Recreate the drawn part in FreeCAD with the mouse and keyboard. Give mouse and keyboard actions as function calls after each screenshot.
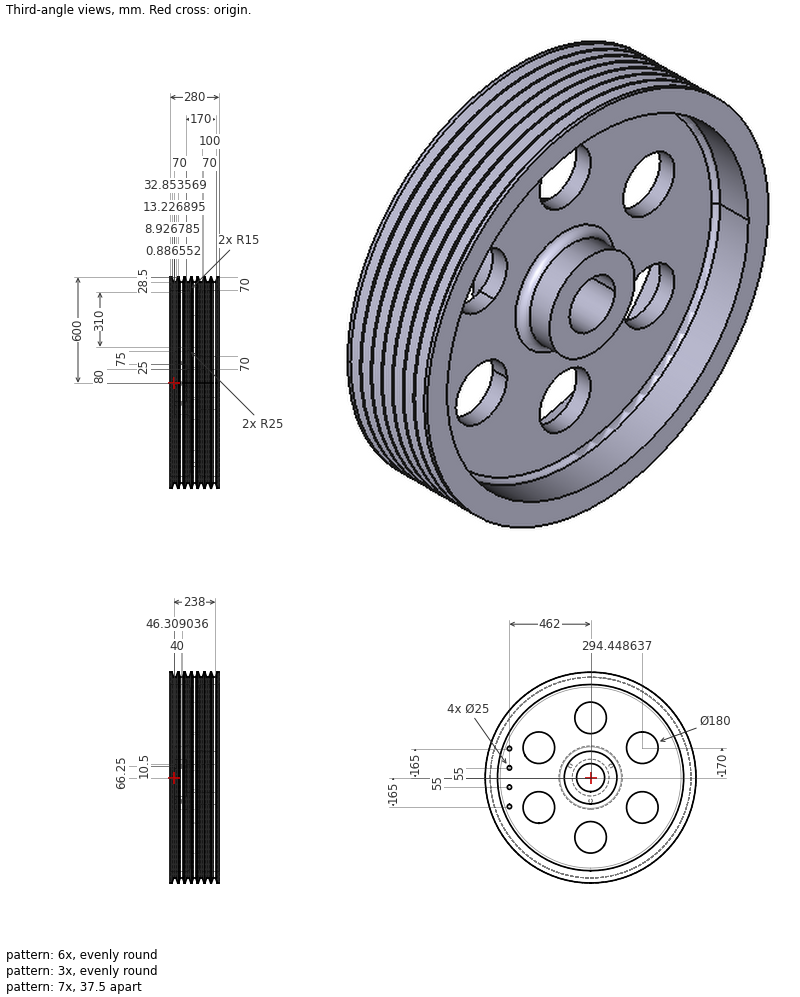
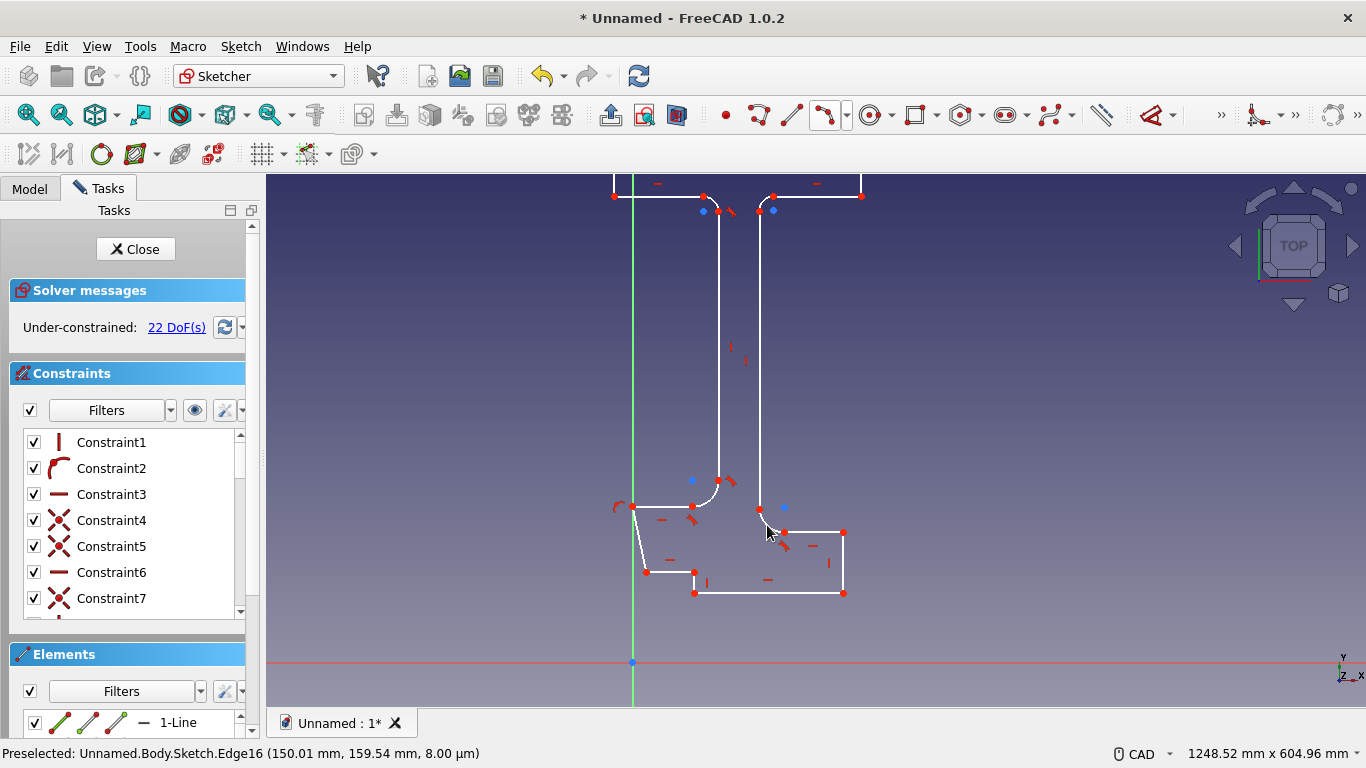
click(760, 420)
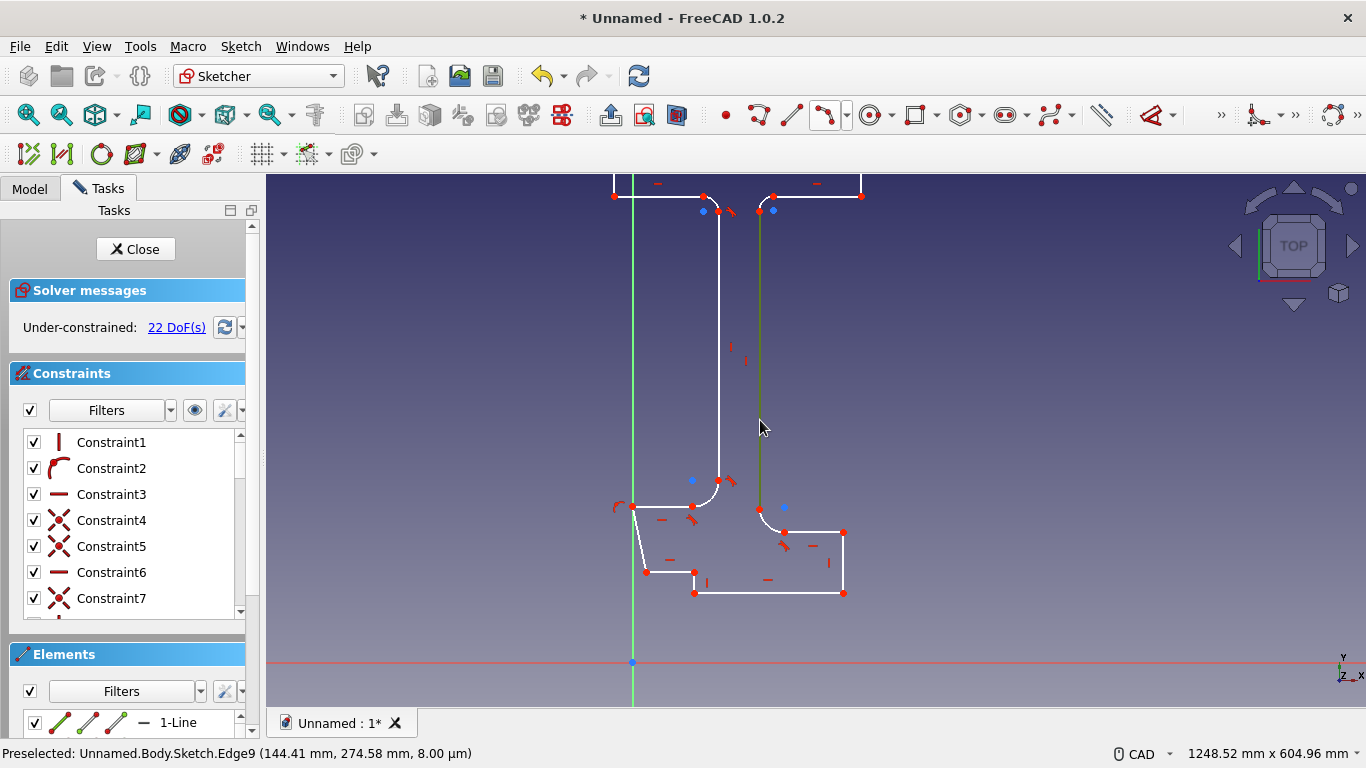
scroll(763, 520, up, 2)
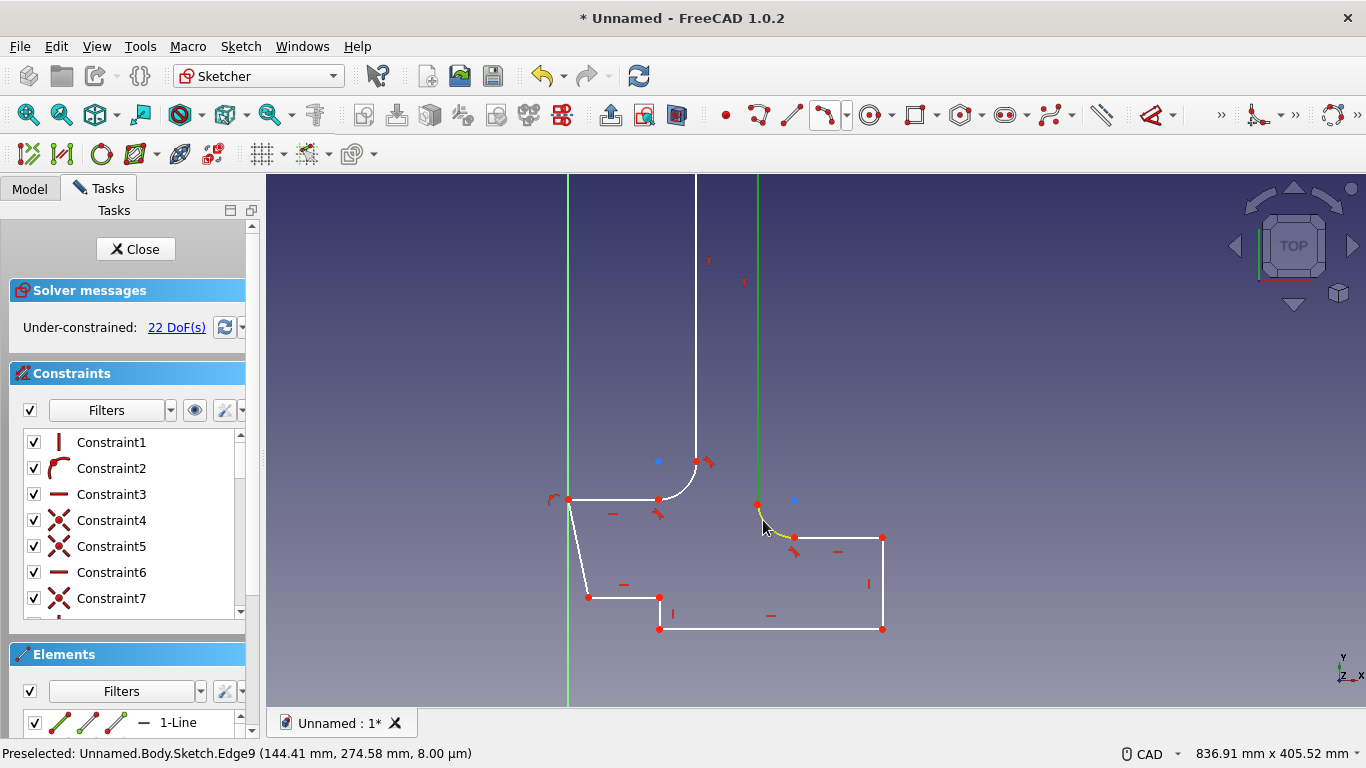
click(763, 520)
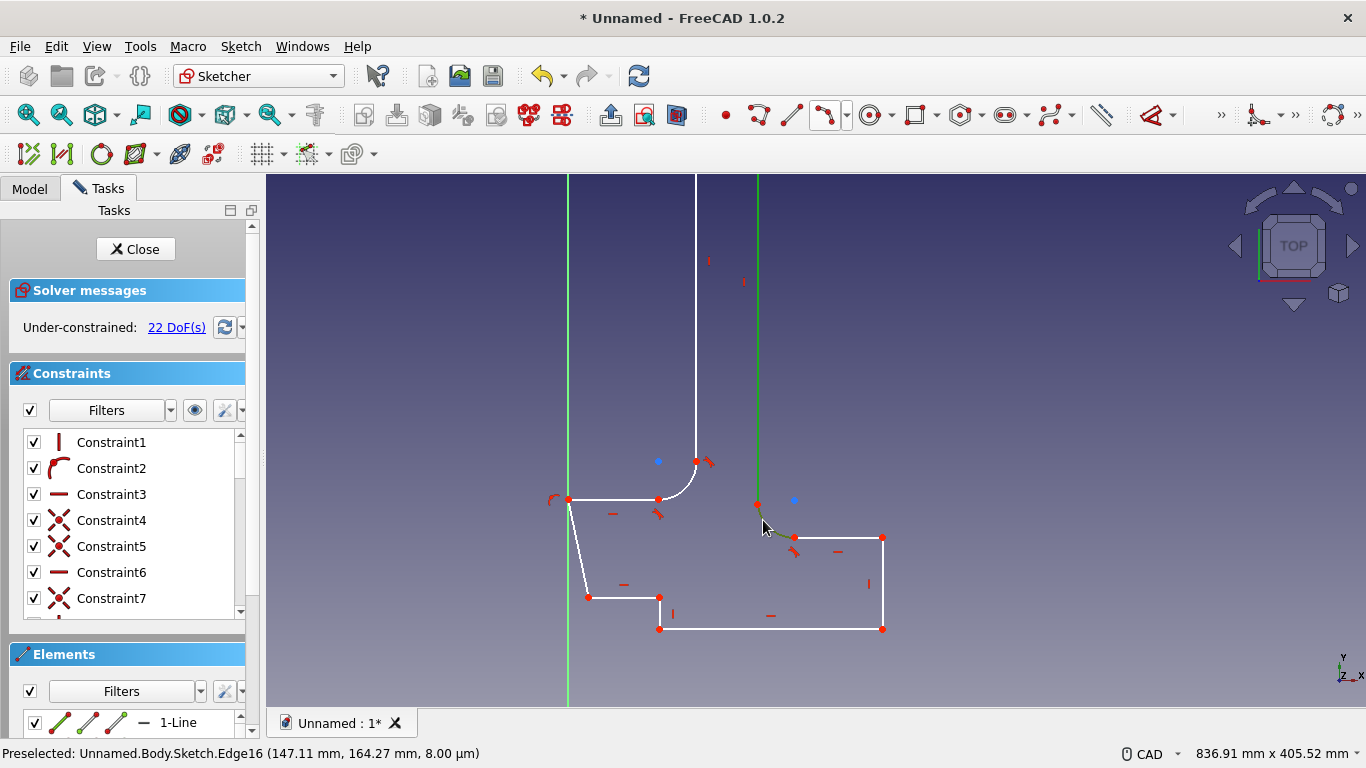
key(t)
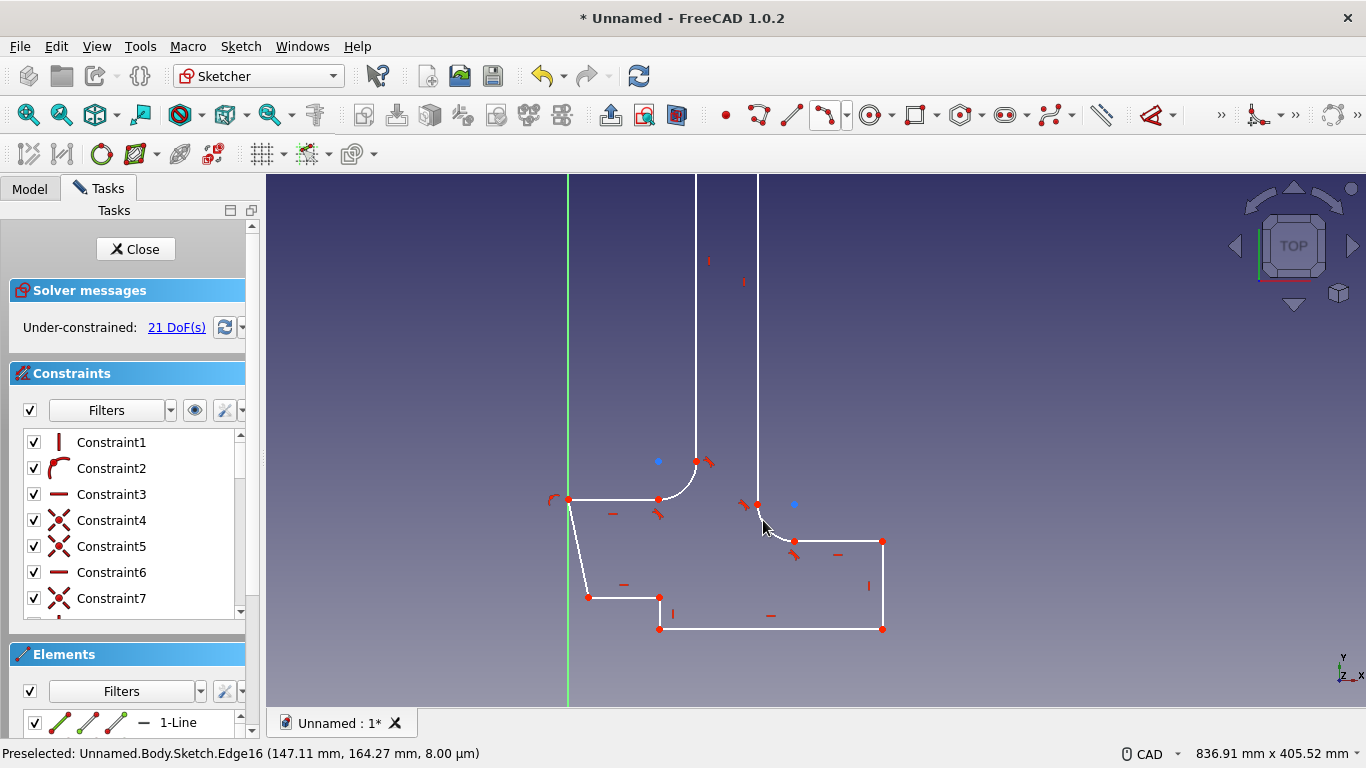
click(758, 371)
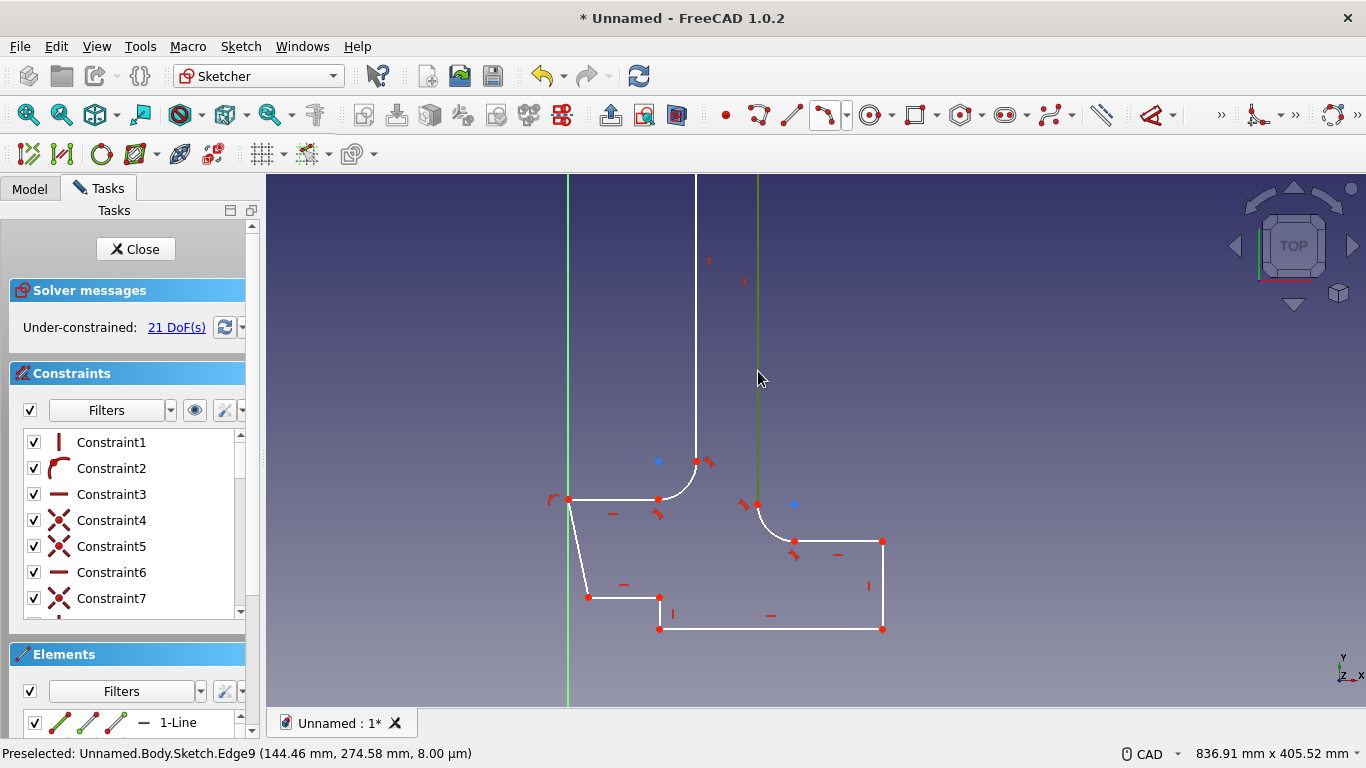
scroll(765, 524, down, 4)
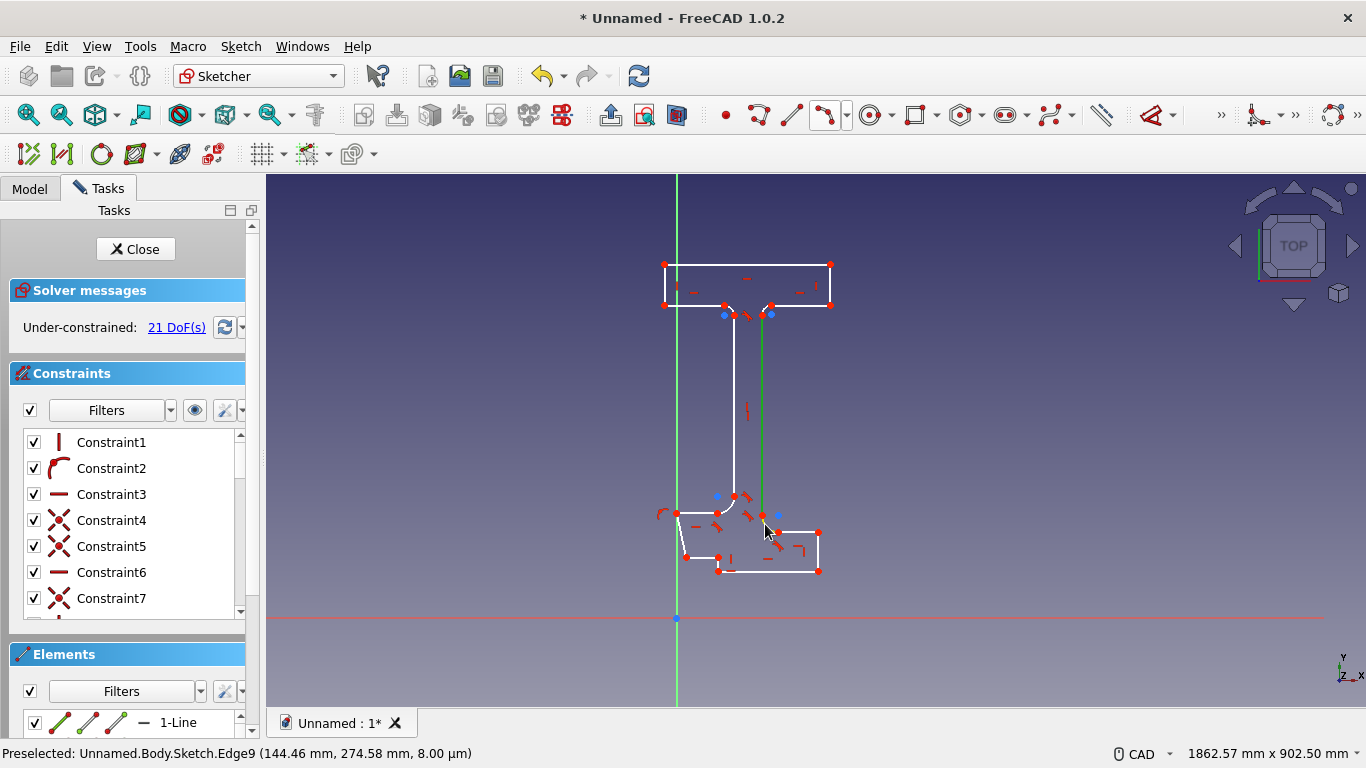
scroll(767, 307, up, 6)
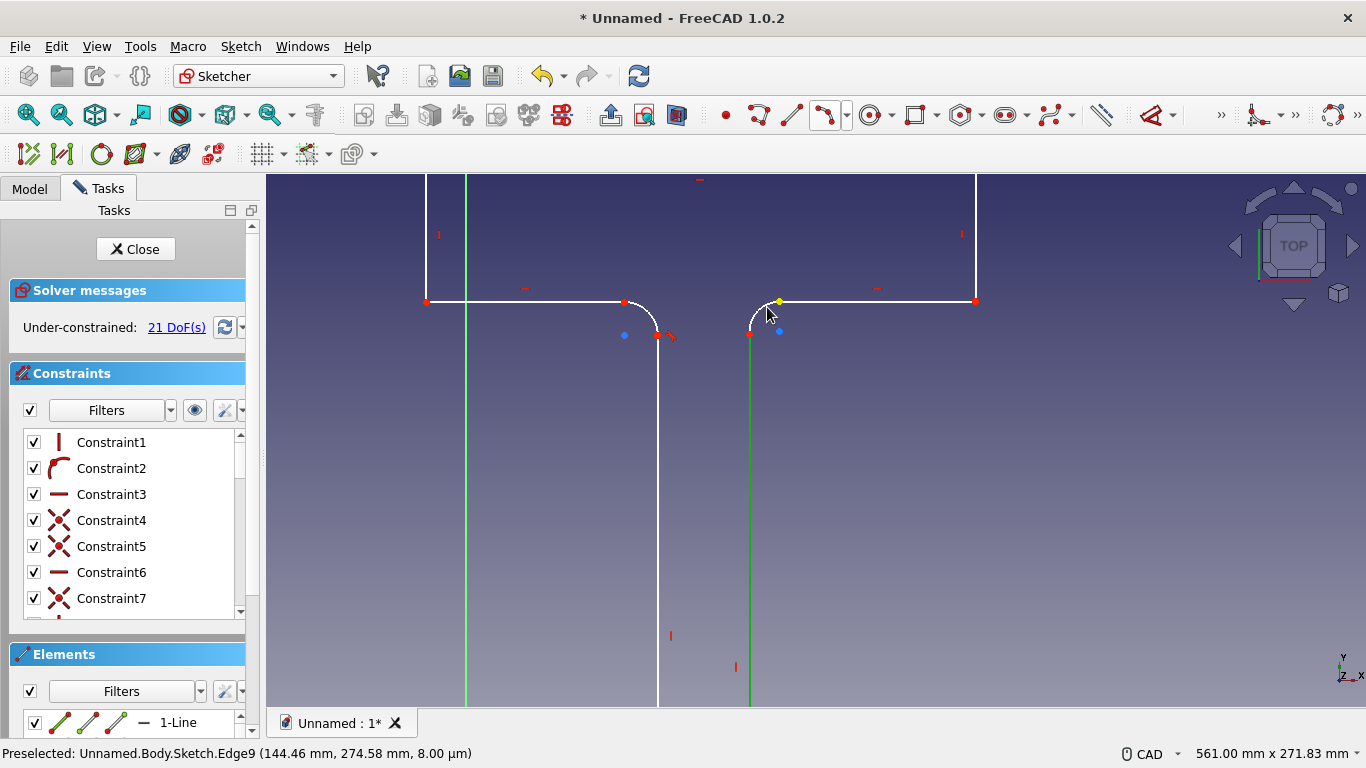
click(765, 305)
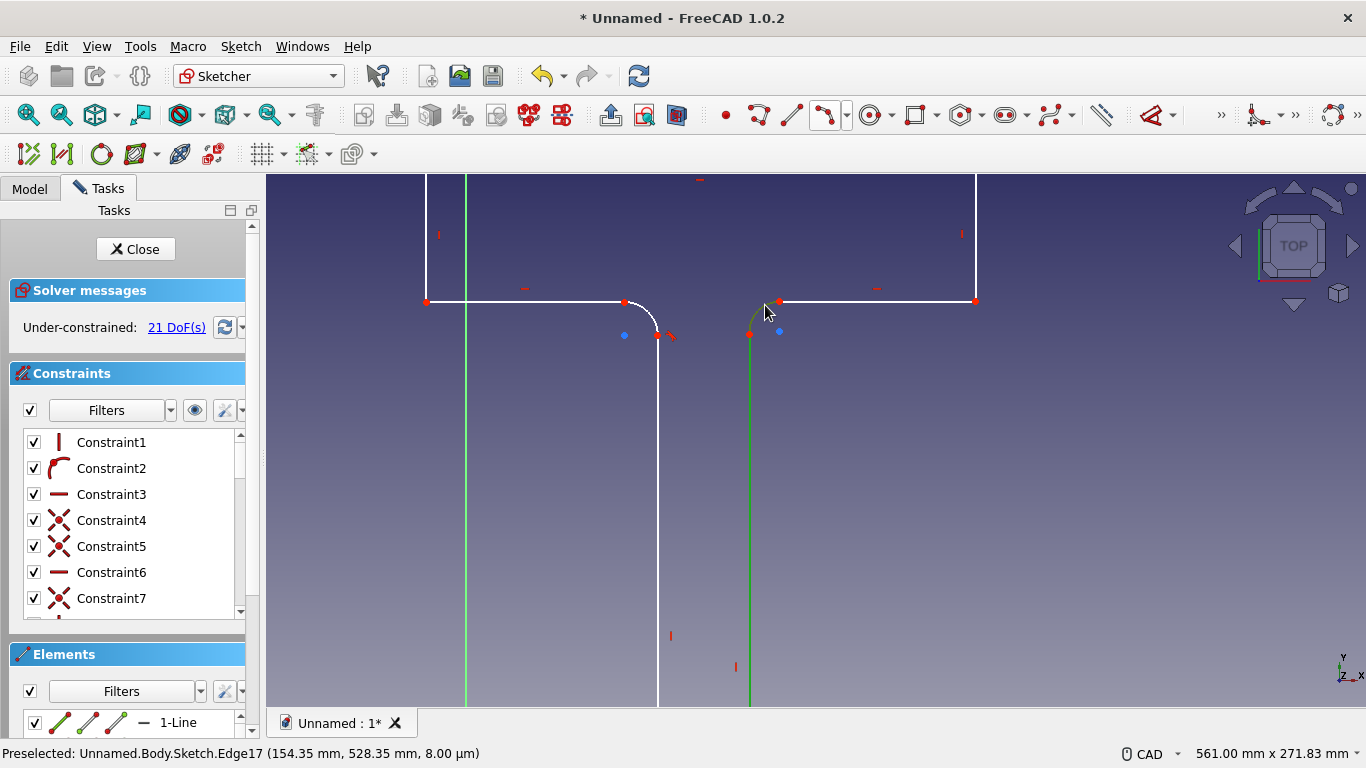
key(t)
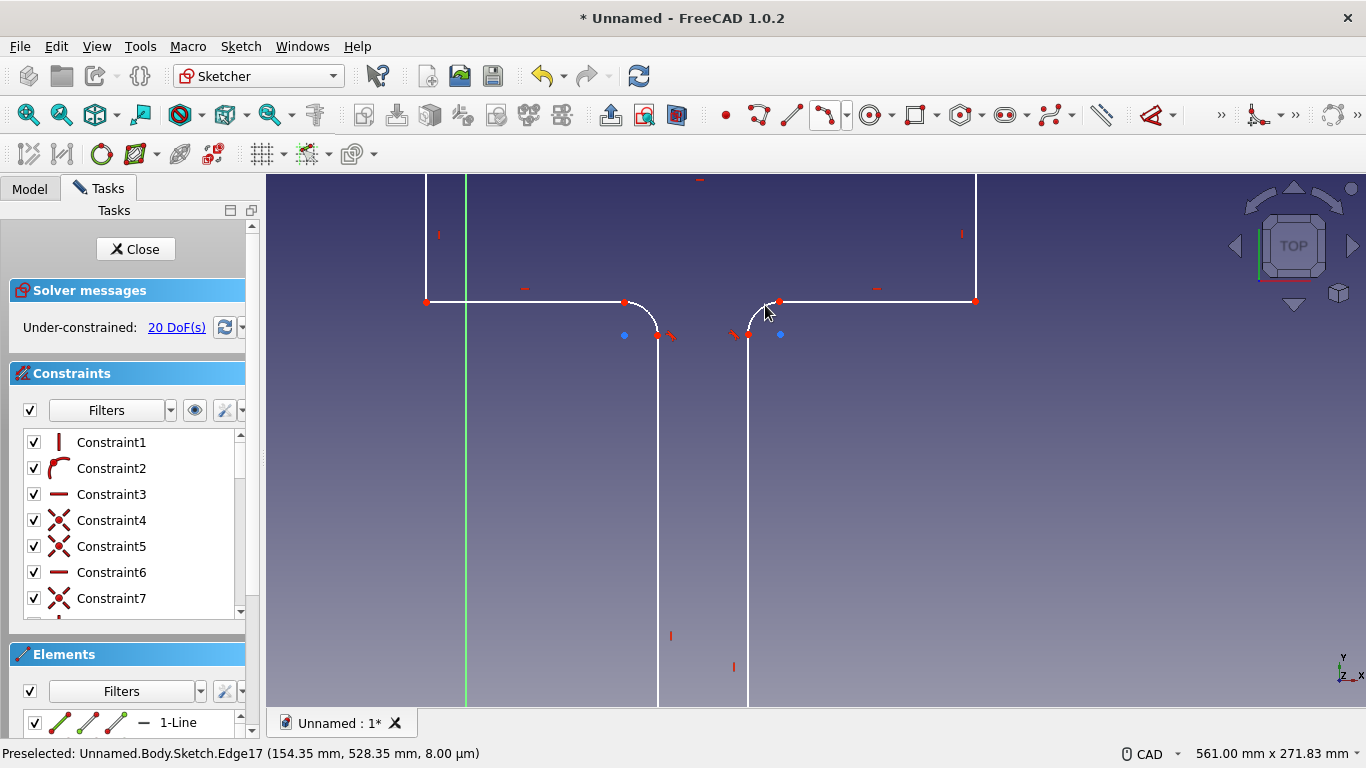
click(839, 302)